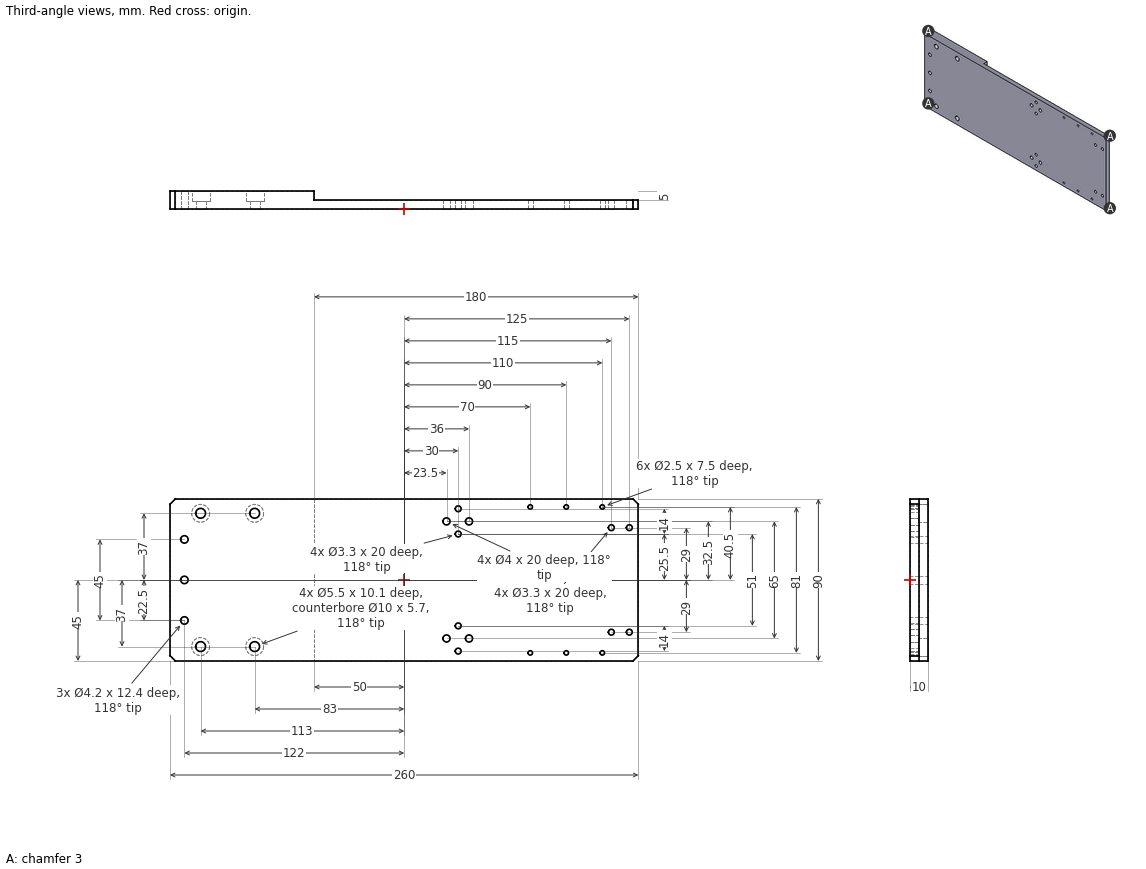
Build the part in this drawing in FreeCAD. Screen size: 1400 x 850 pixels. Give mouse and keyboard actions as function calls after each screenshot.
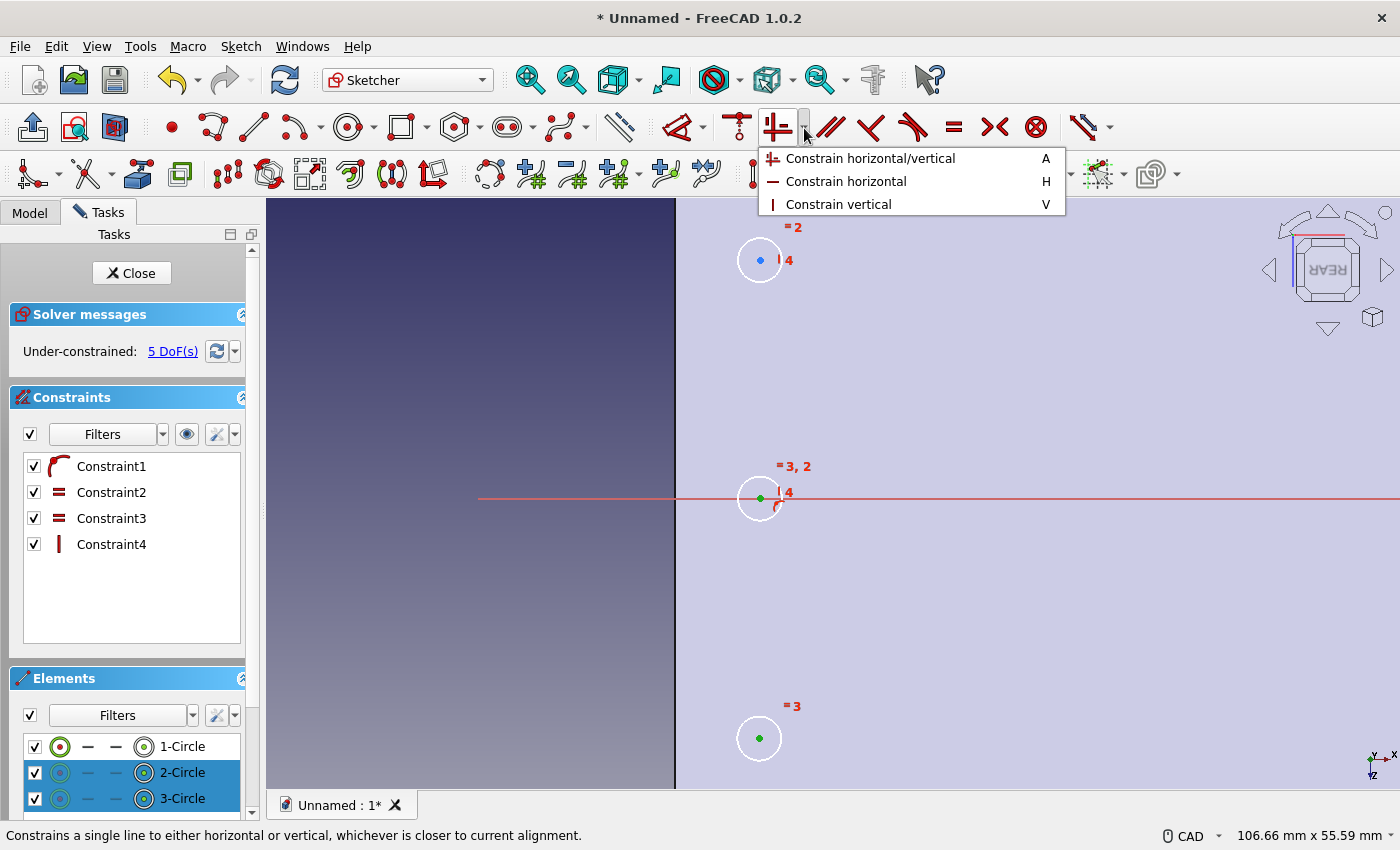
click(912, 204)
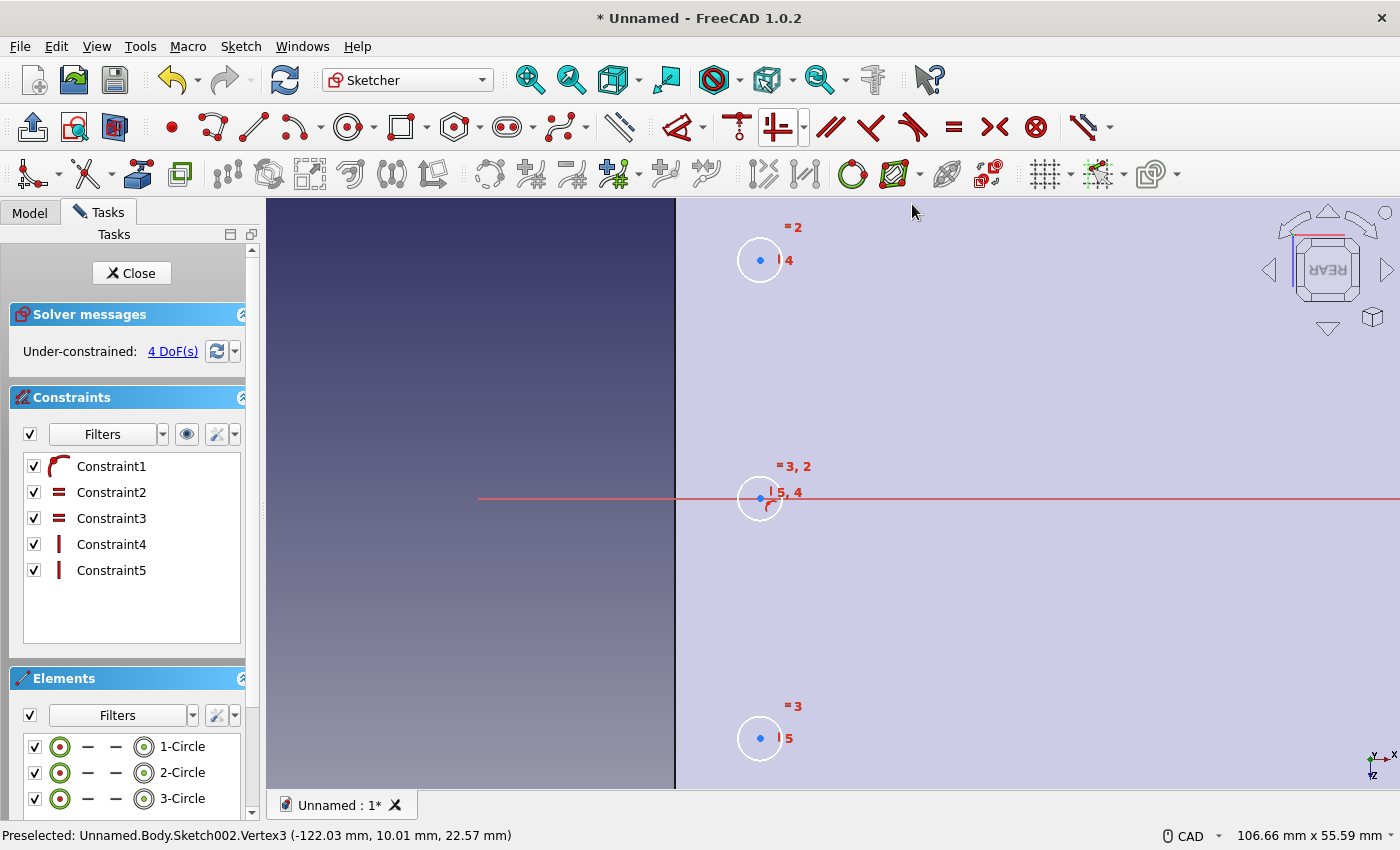
click(676, 128)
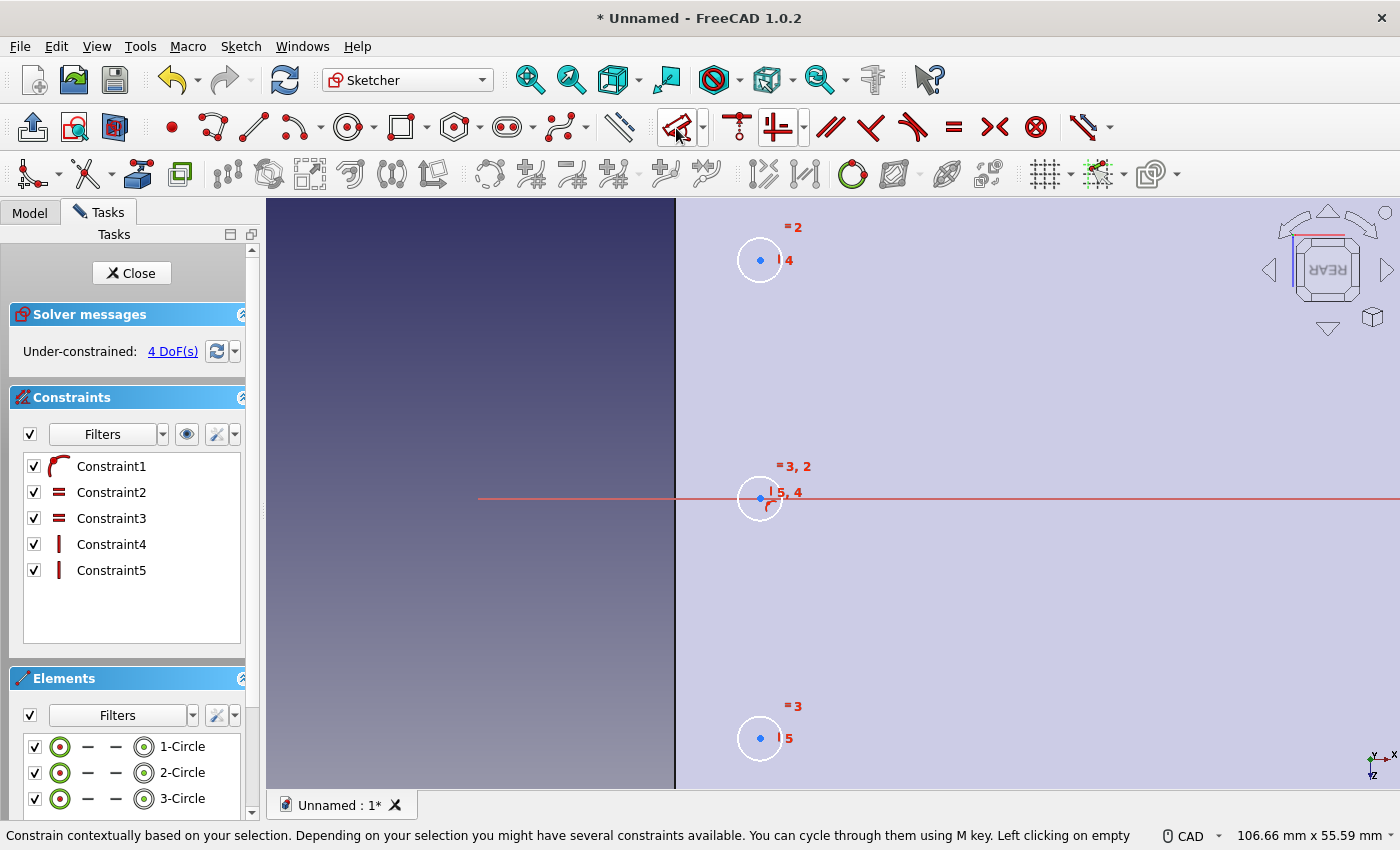
click(776, 245)
click(812, 246)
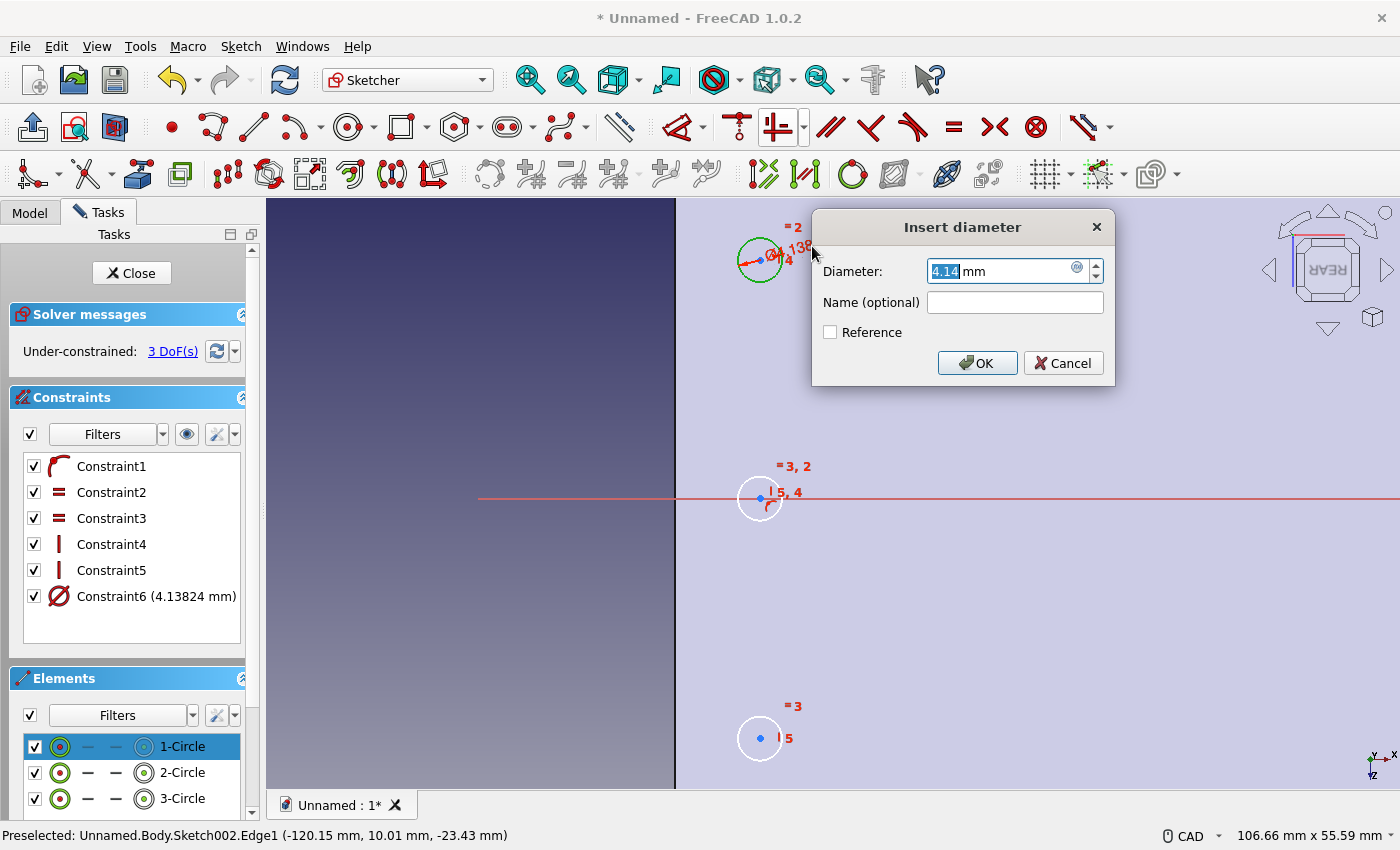
text(4.2)
key(Return)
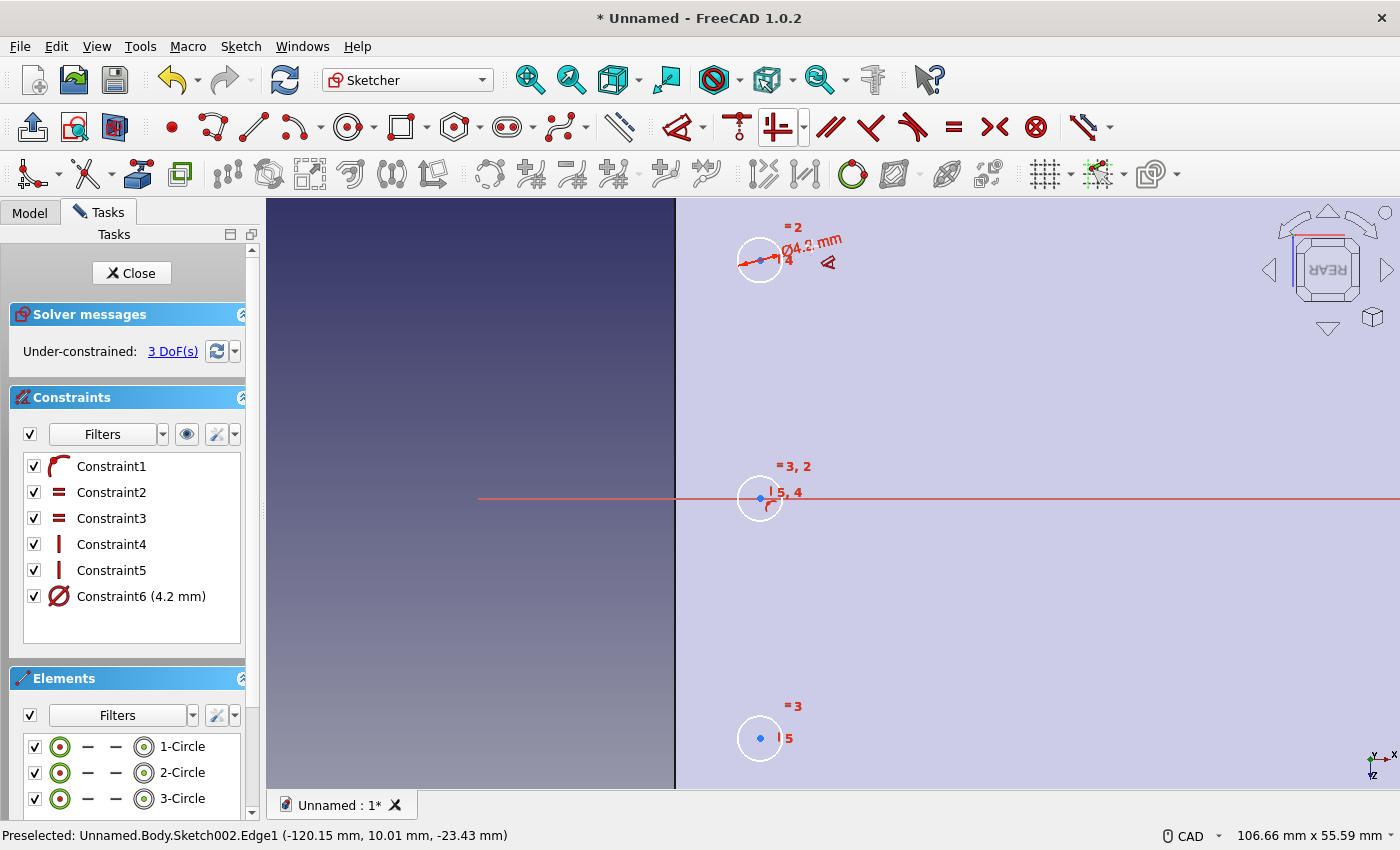
click(760, 260)
click(998, 226)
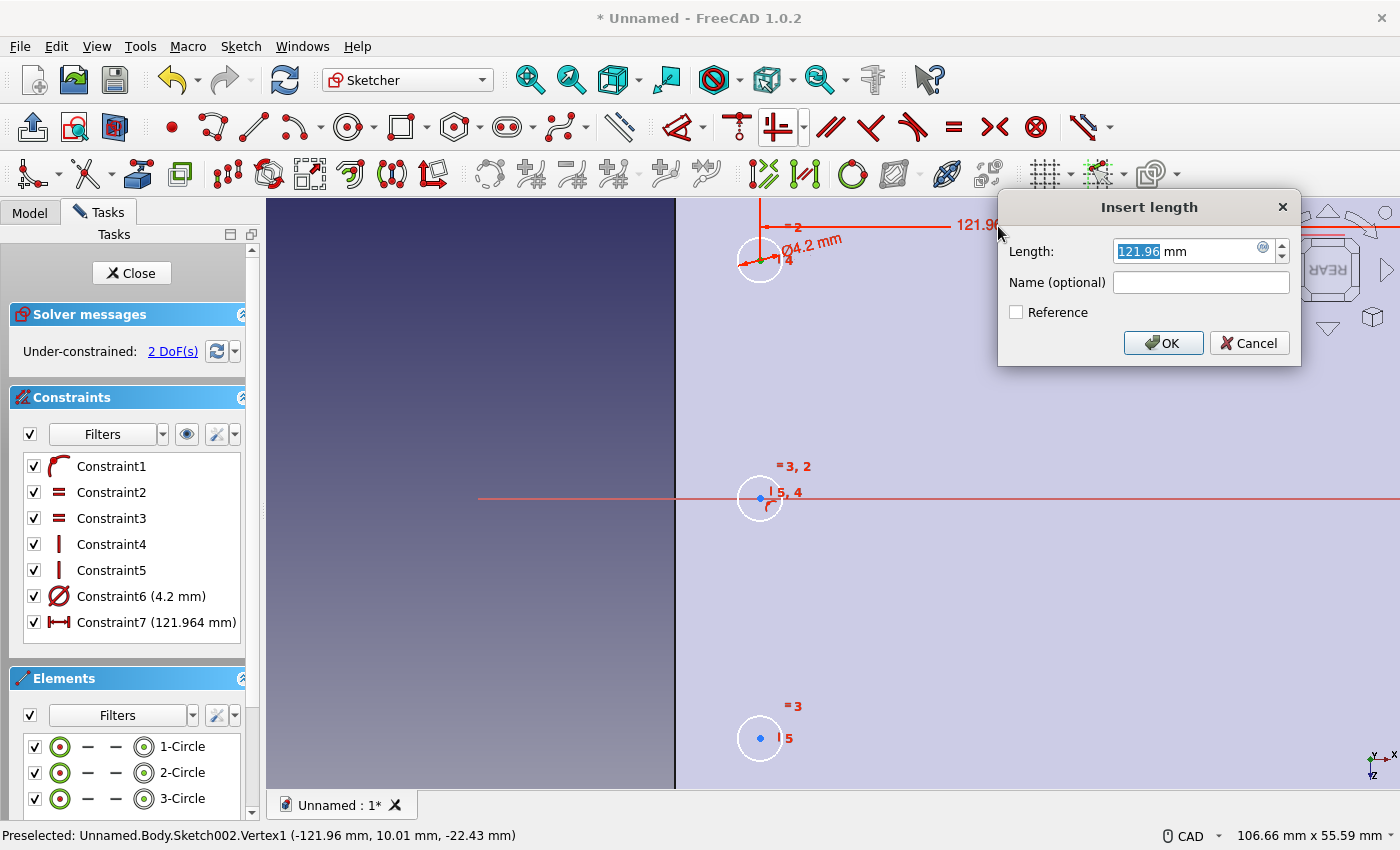
text(122)
key(Return)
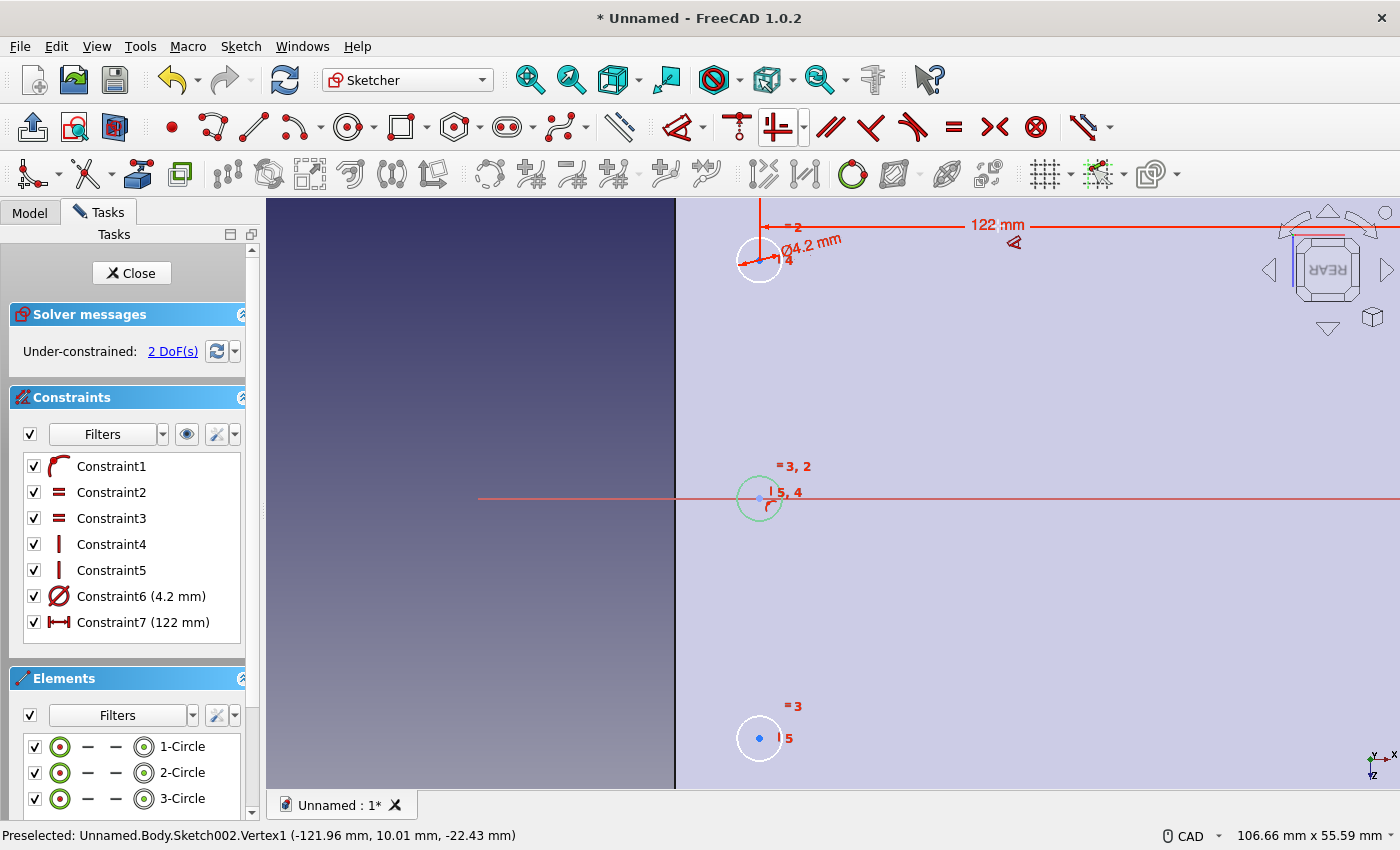
click(760, 260)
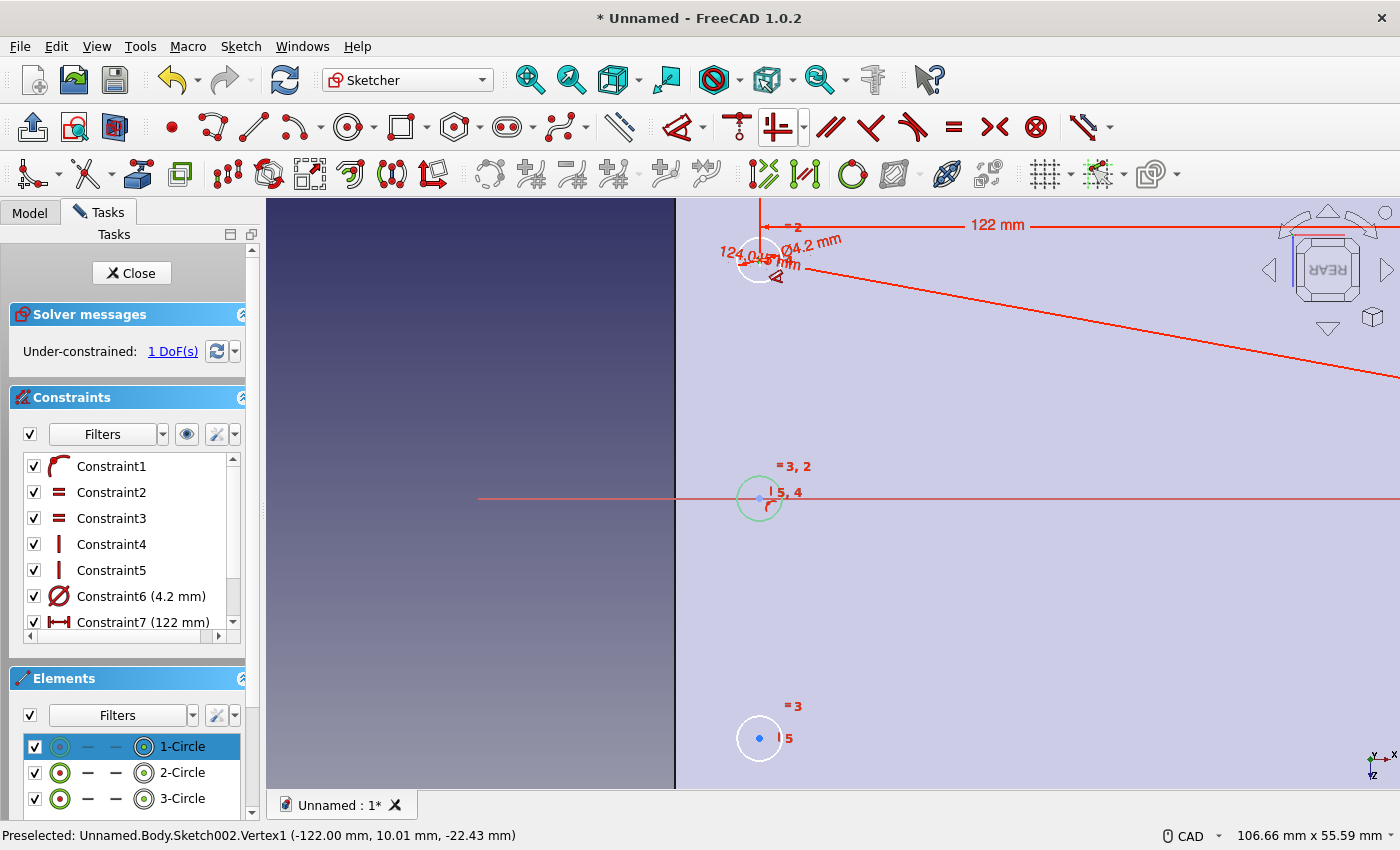
click(760, 739)
click(794, 389)